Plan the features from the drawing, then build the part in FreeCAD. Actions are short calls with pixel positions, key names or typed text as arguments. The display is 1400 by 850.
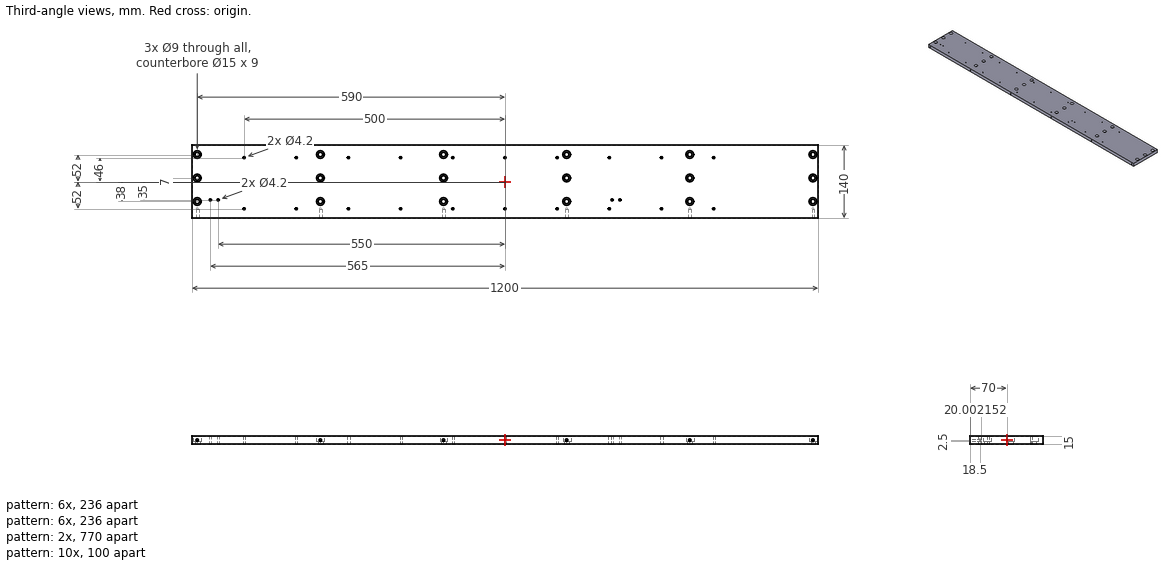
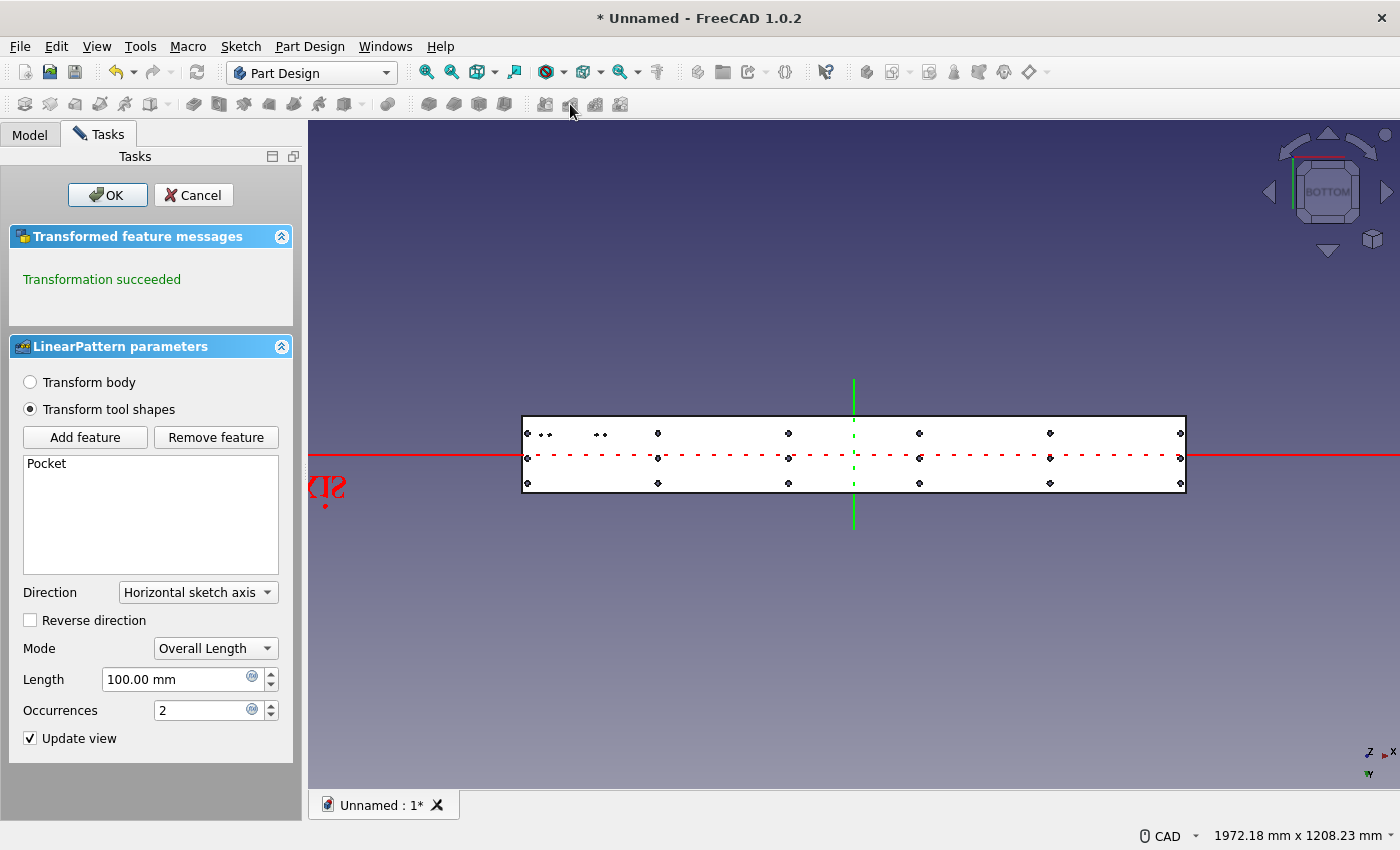
click(199, 592)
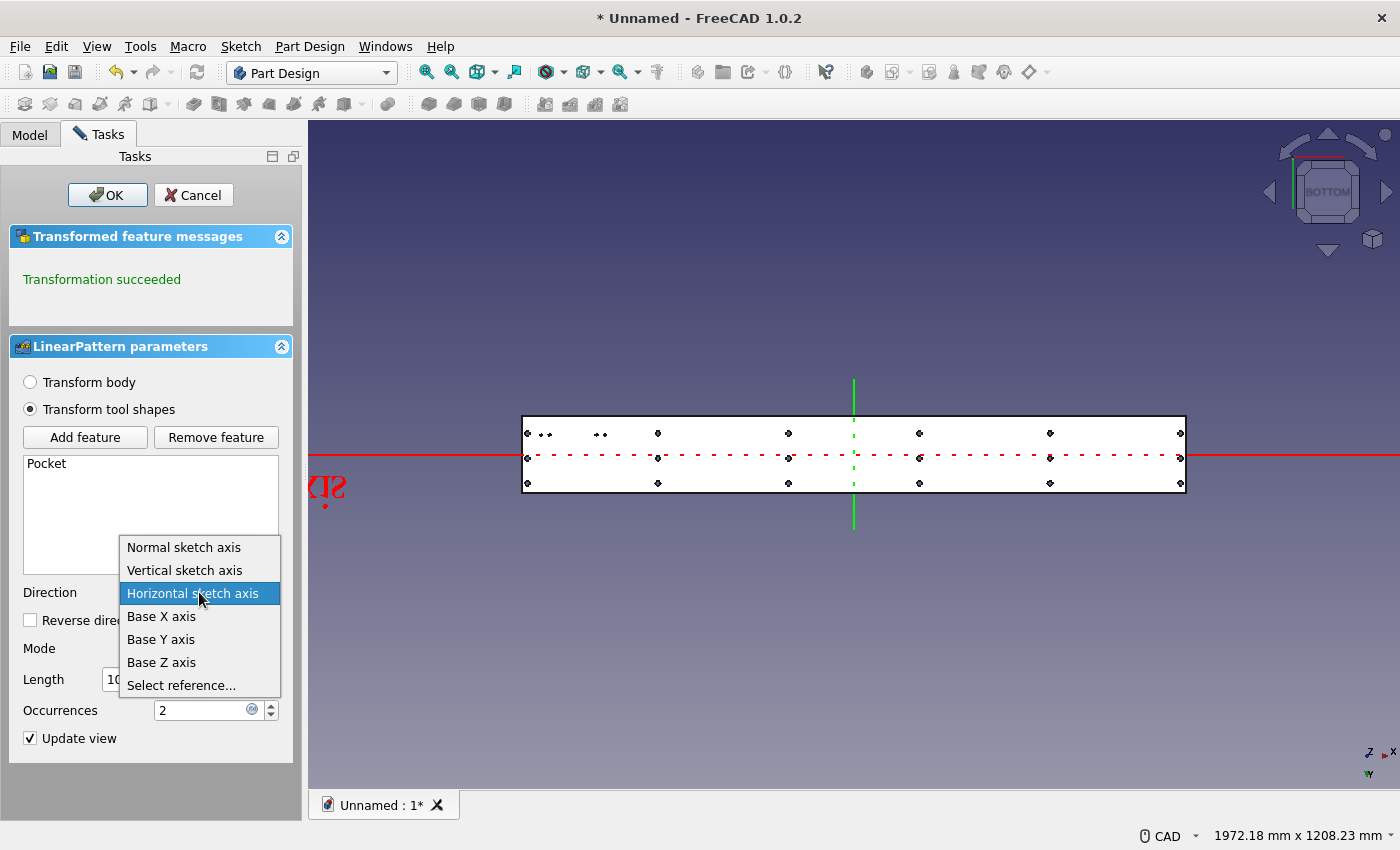
click(198, 616)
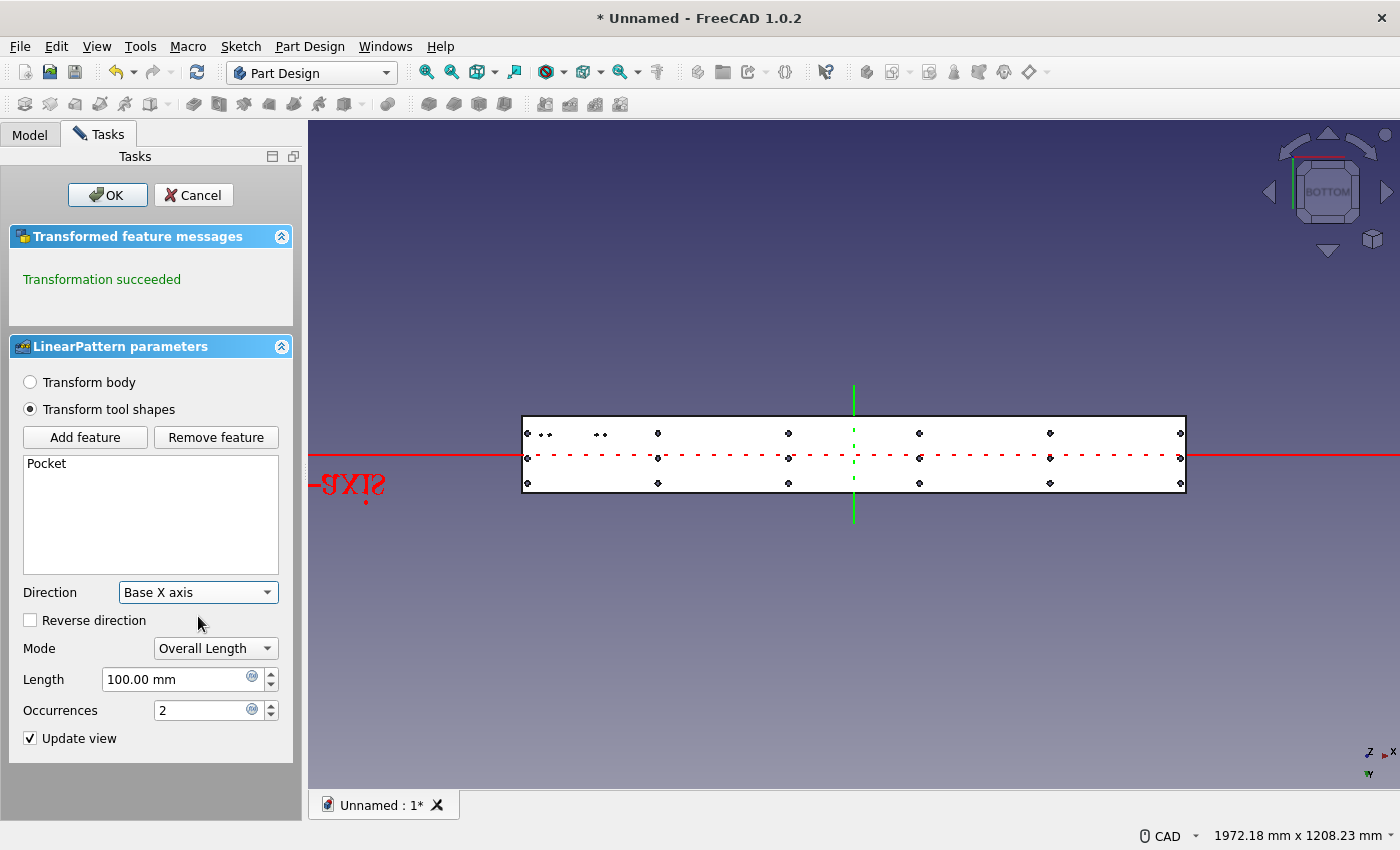
click(216, 648)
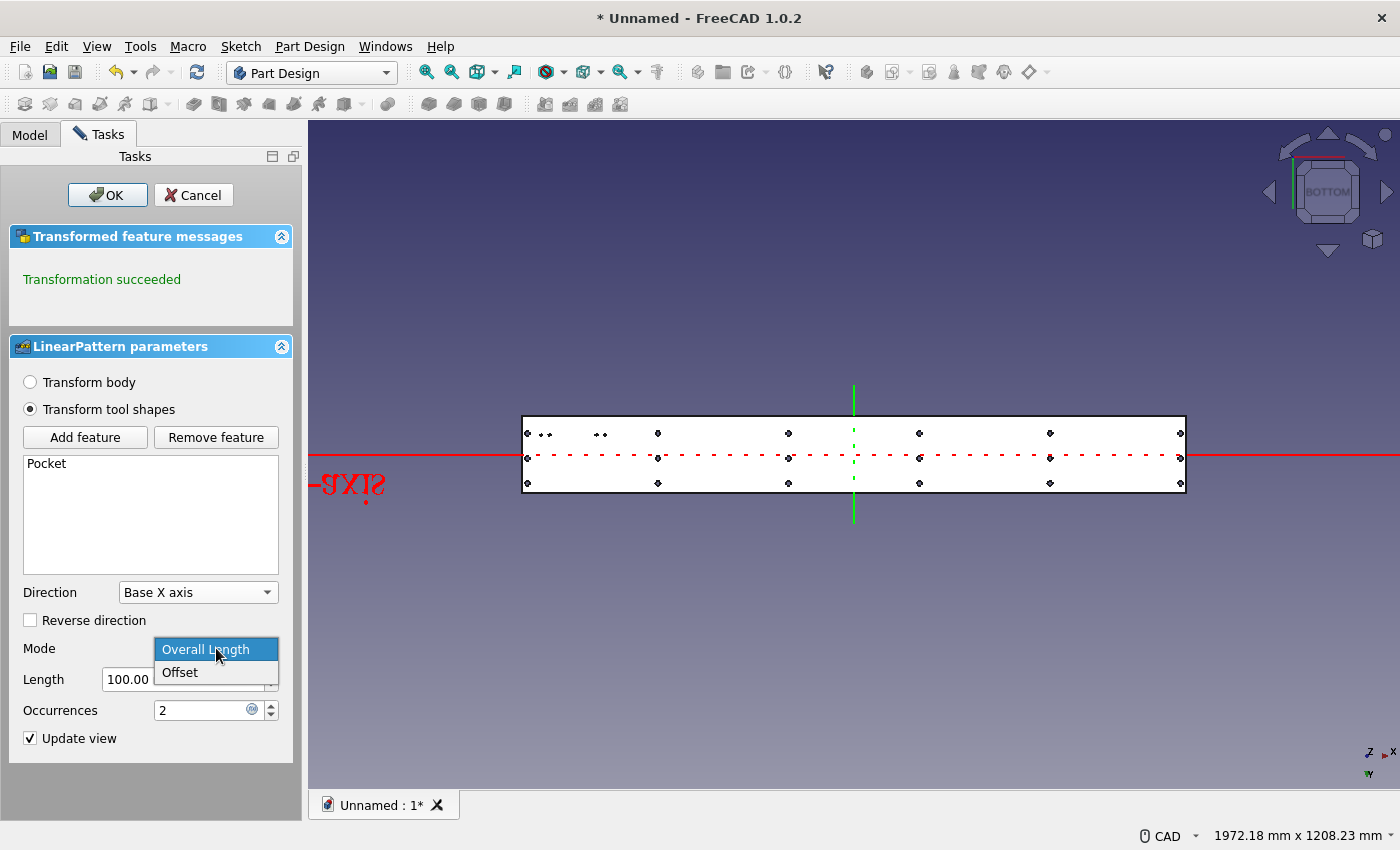
click(214, 672)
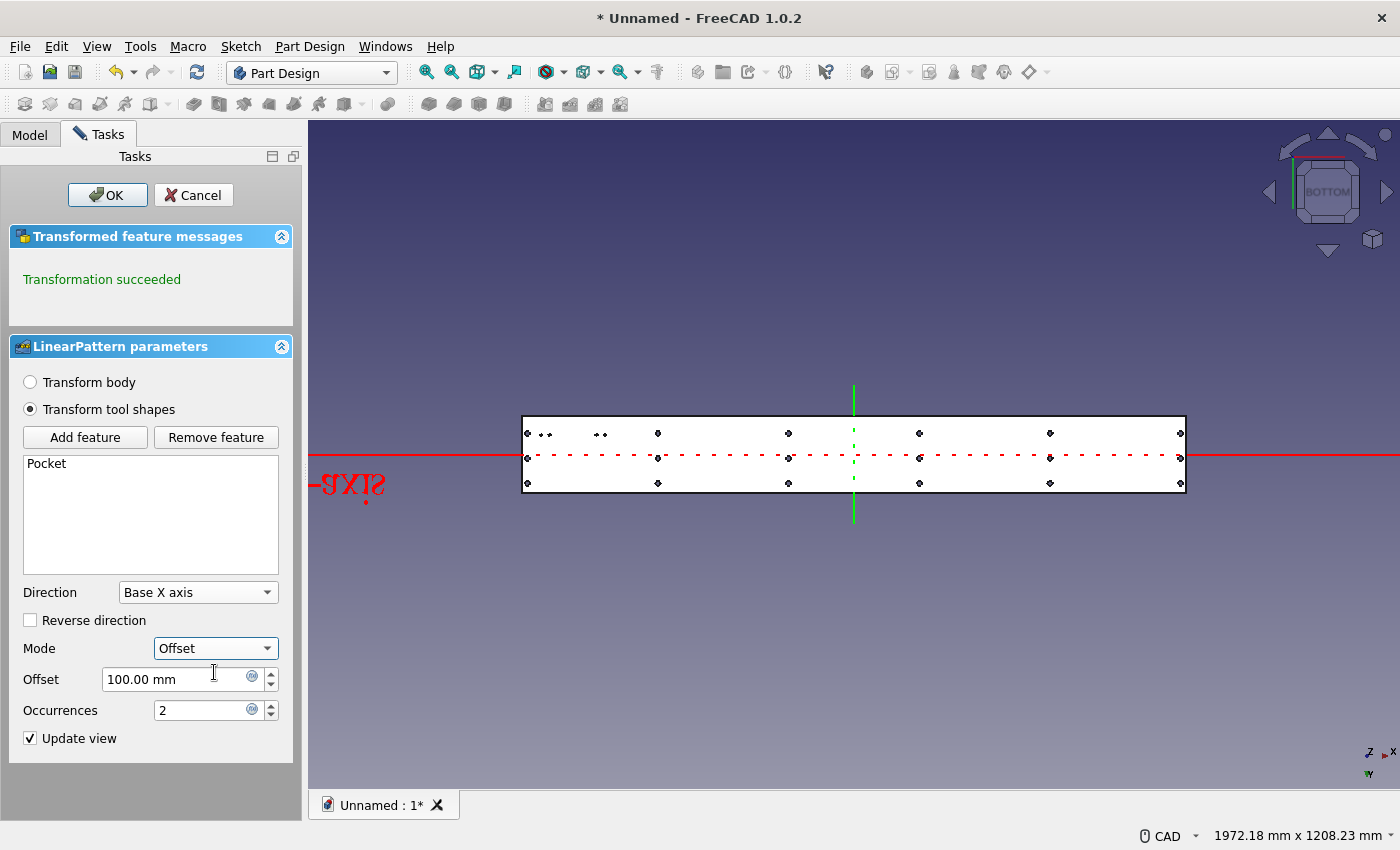
triple_click(184, 680)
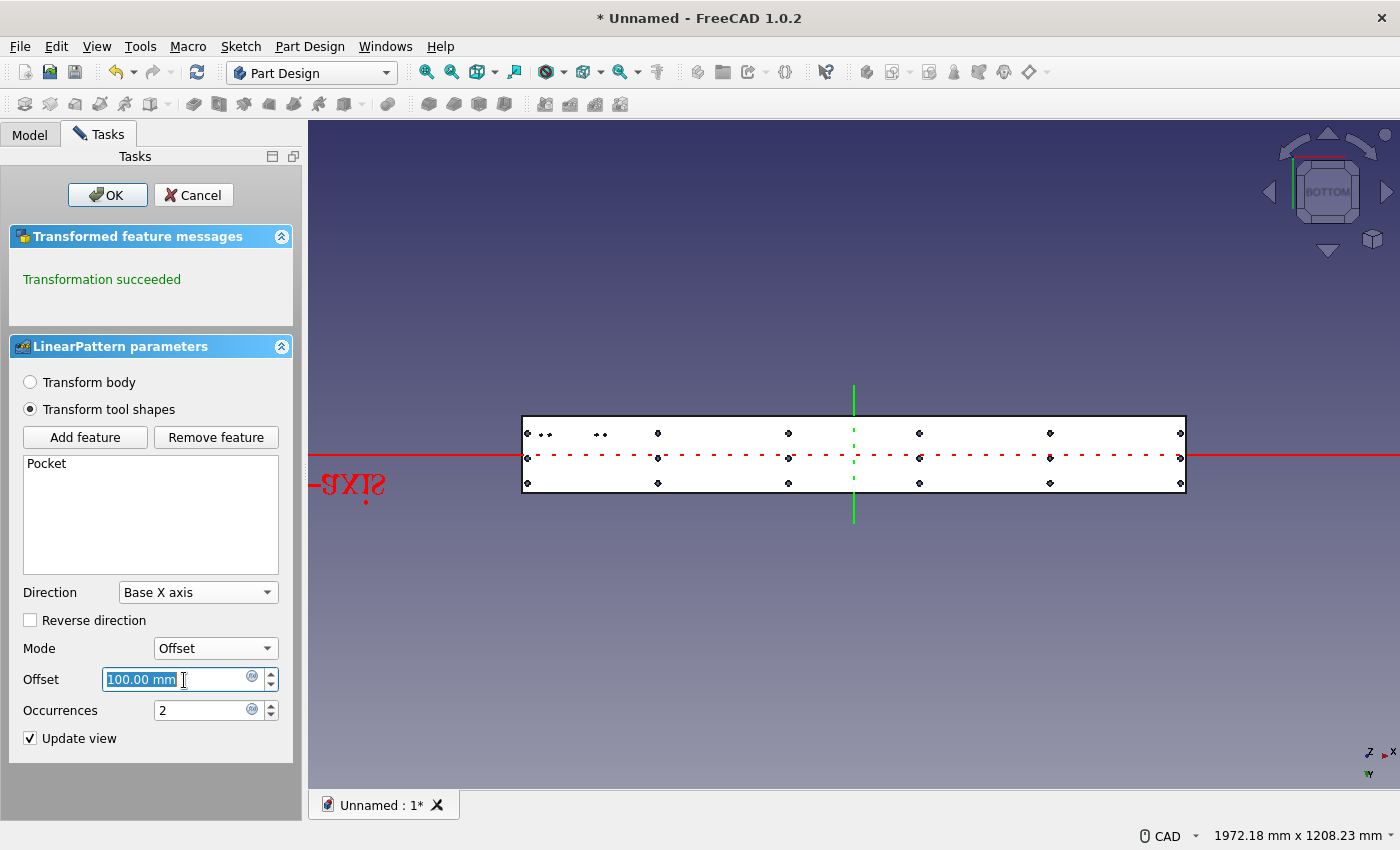
text(770)
key(Tab)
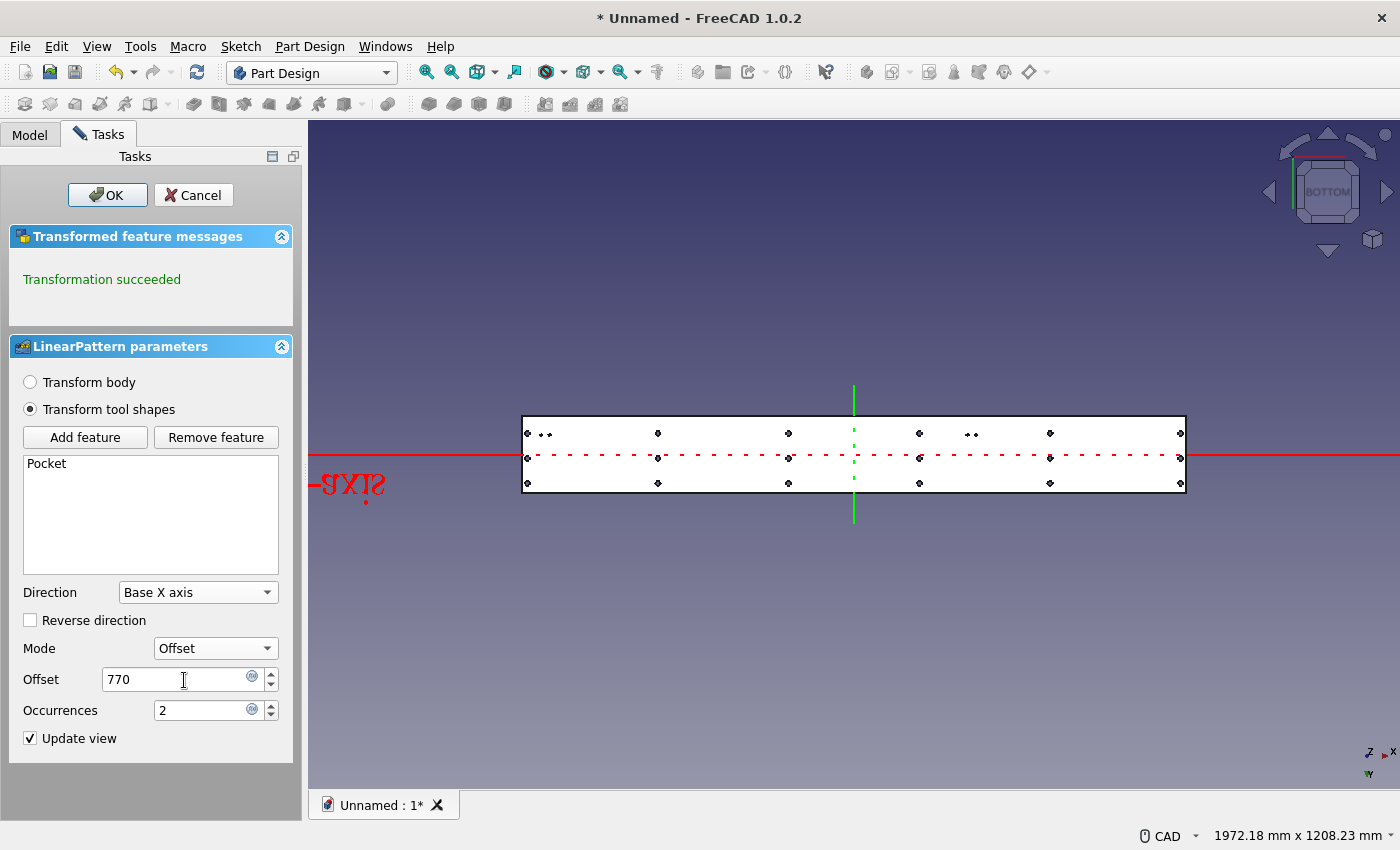
triple_click(210, 710)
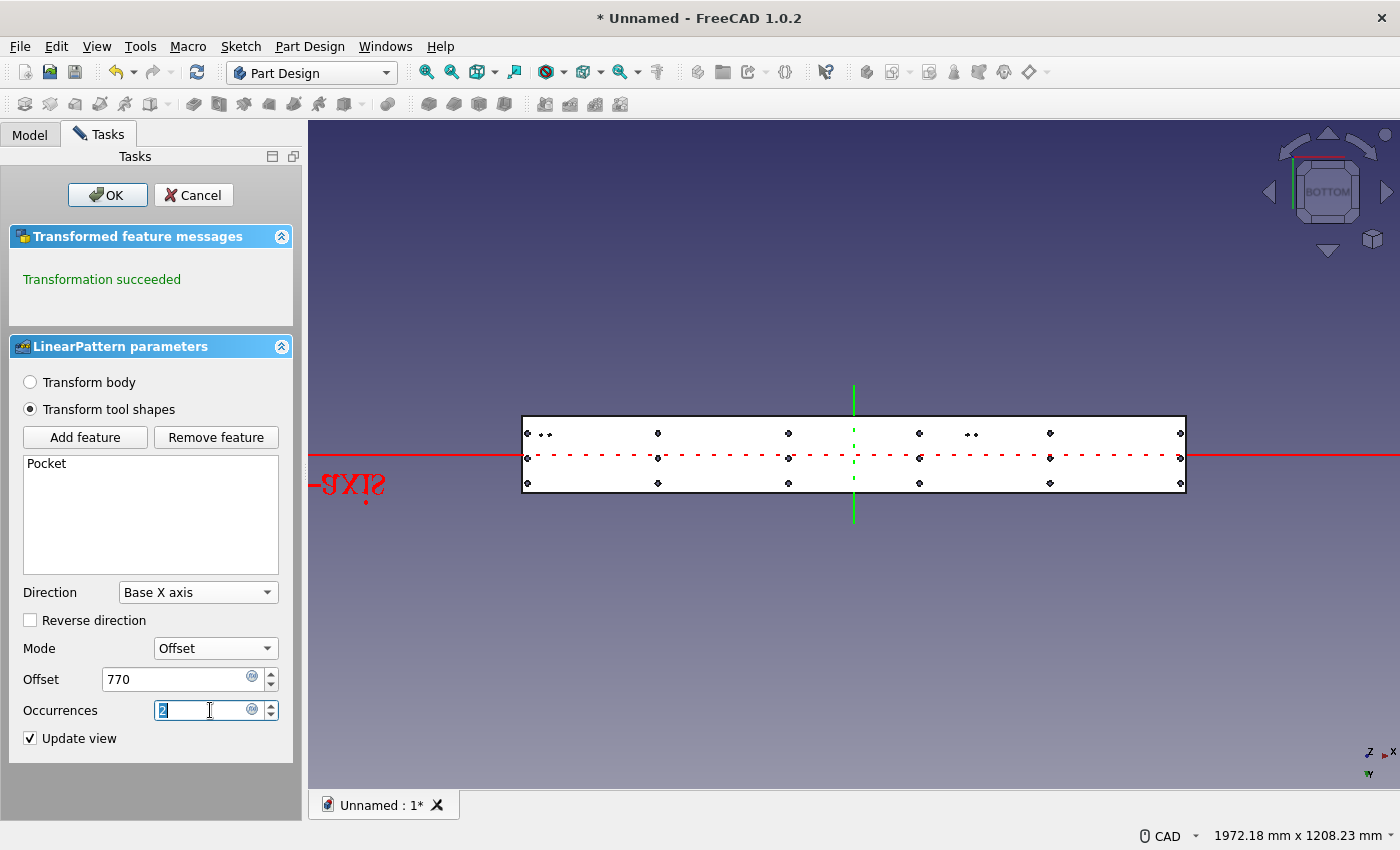
text(2)
key(Tab)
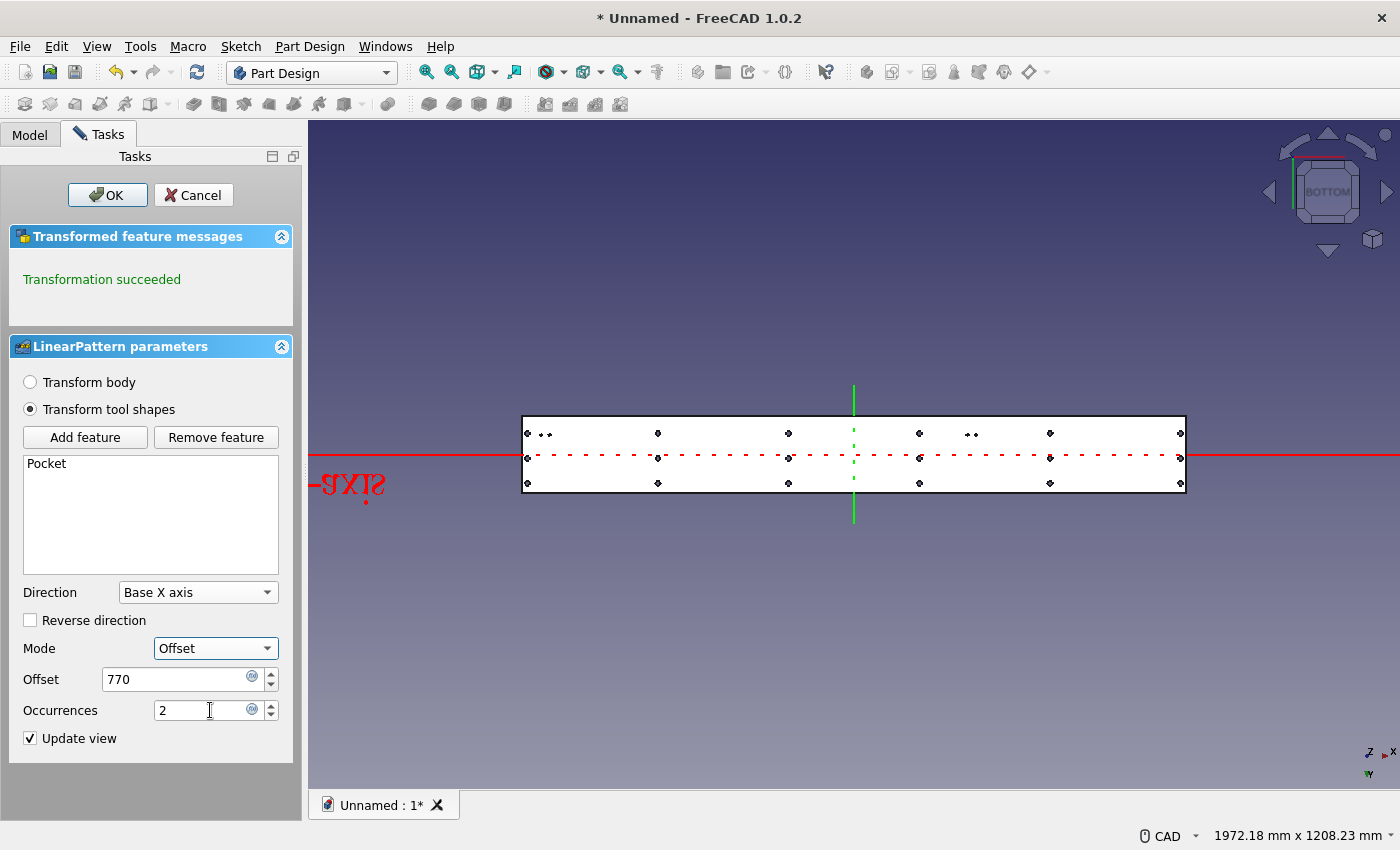
click(108, 195)